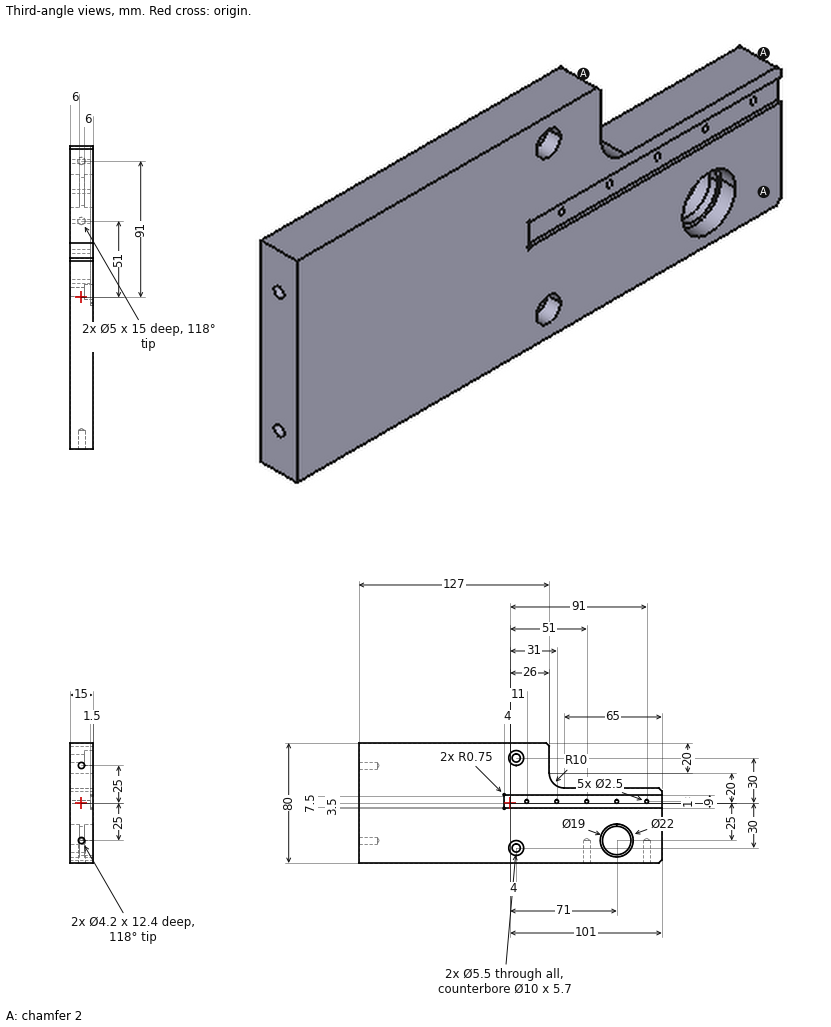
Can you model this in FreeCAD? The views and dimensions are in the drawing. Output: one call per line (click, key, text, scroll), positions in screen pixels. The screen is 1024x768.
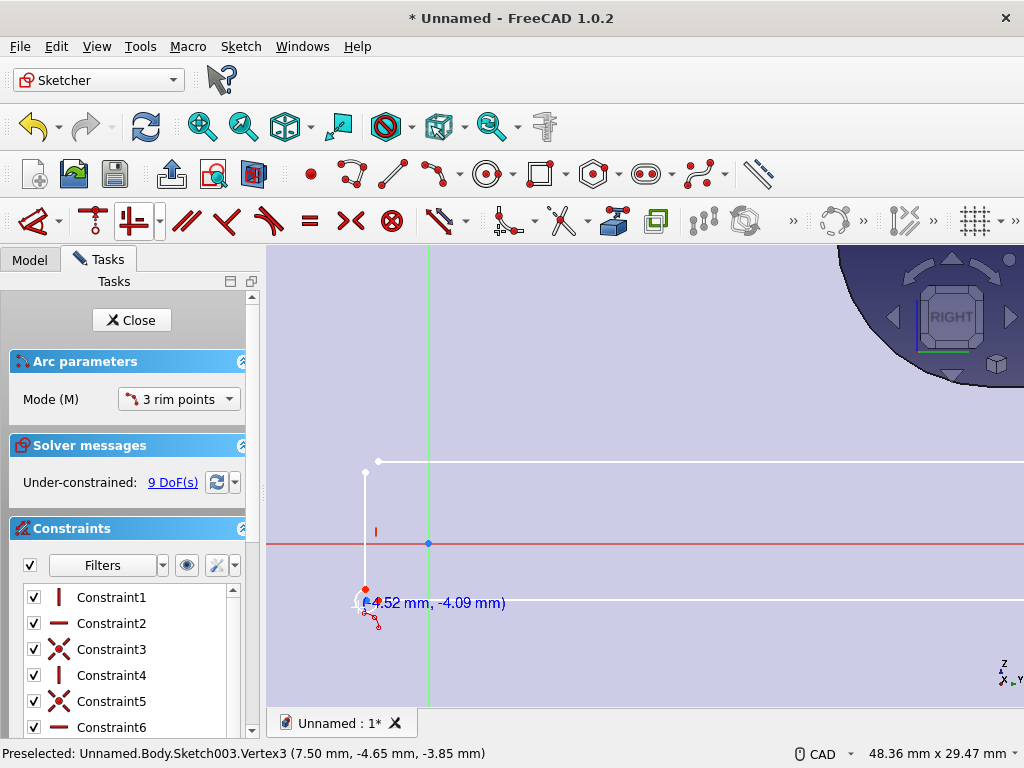
click(378, 462)
click(365, 473)
click(358, 449)
key(Escape)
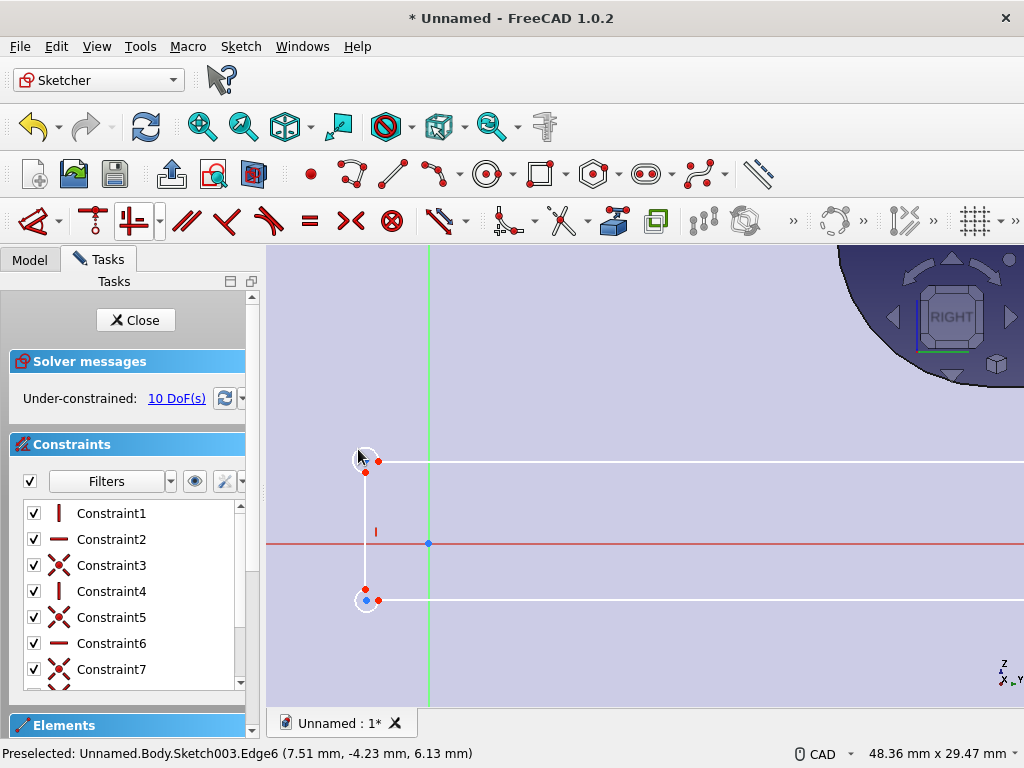
click(355, 600)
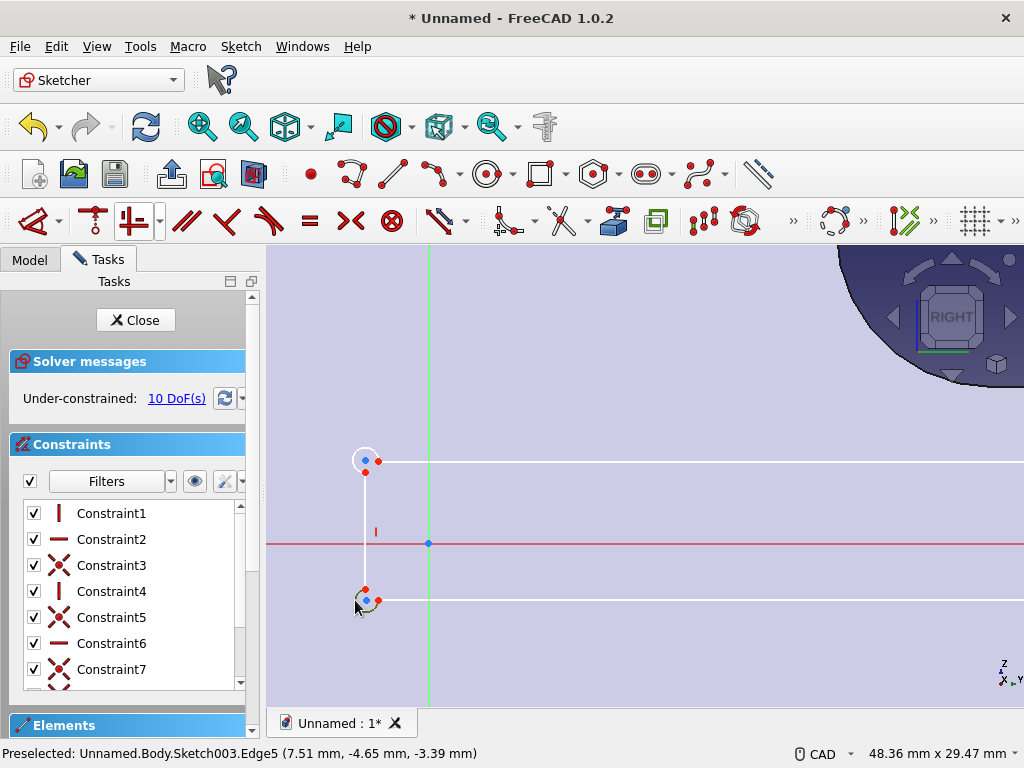
click(369, 448)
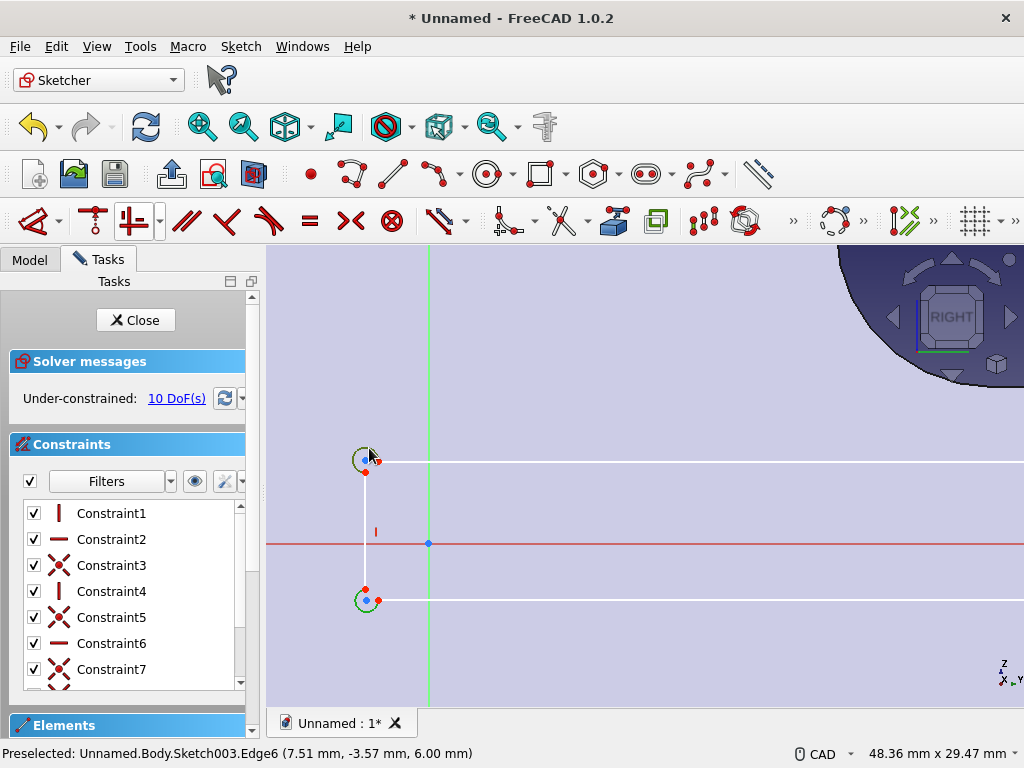
click(310, 222)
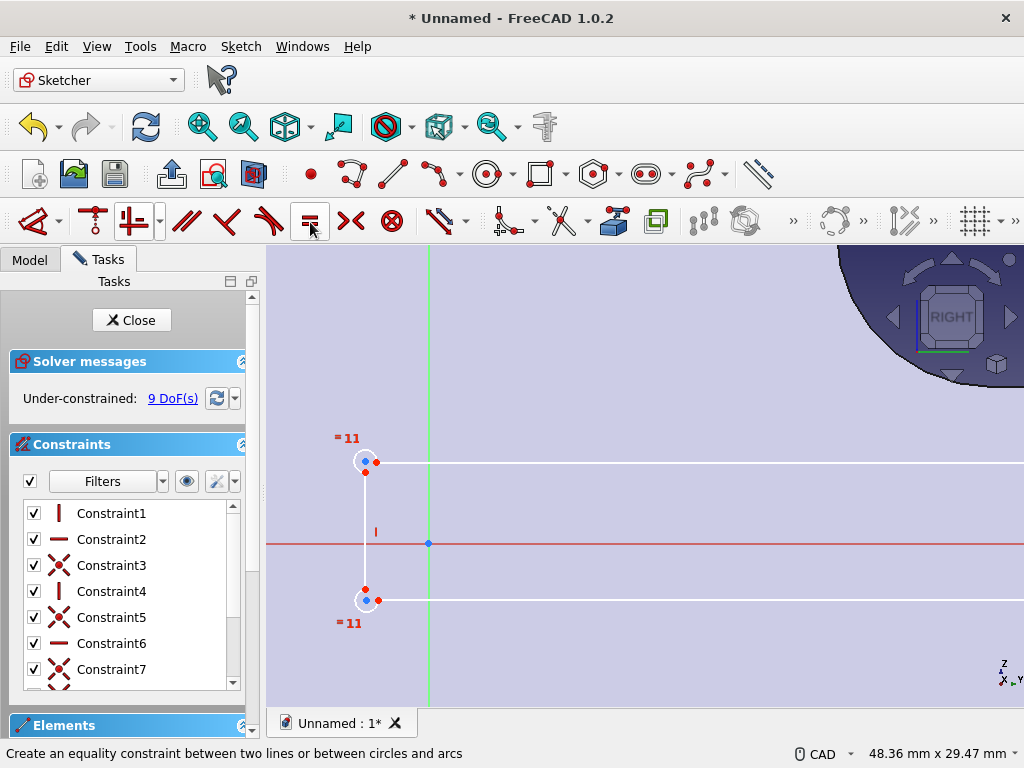
key(d)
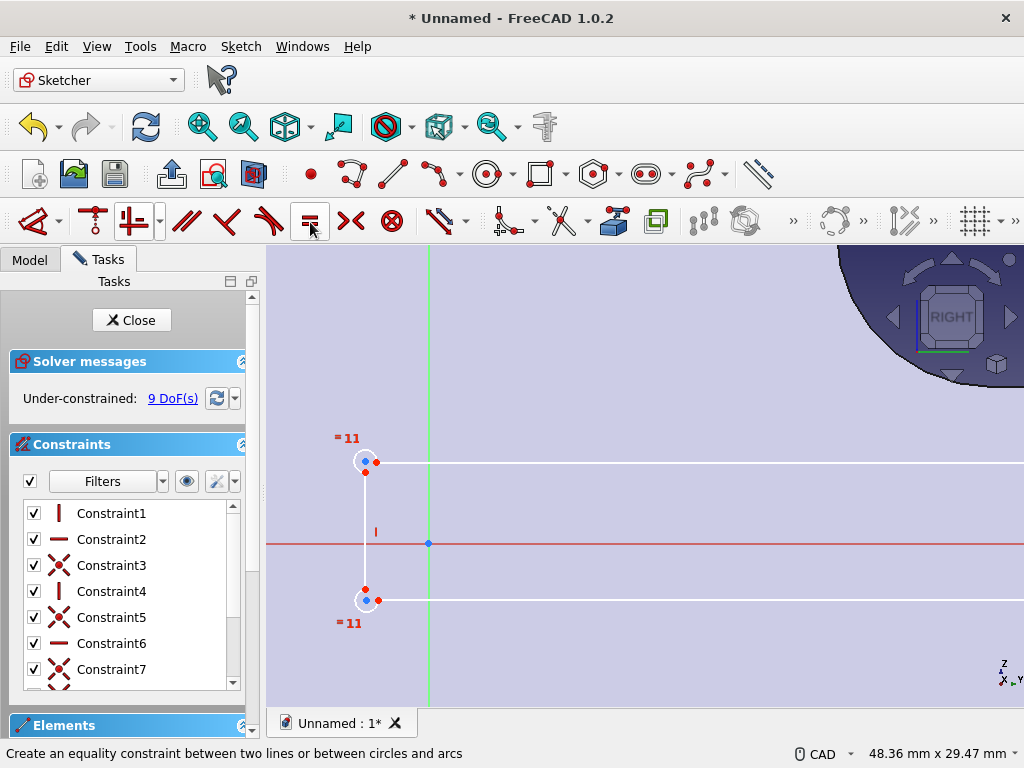
scroll(355, 600, up, 7)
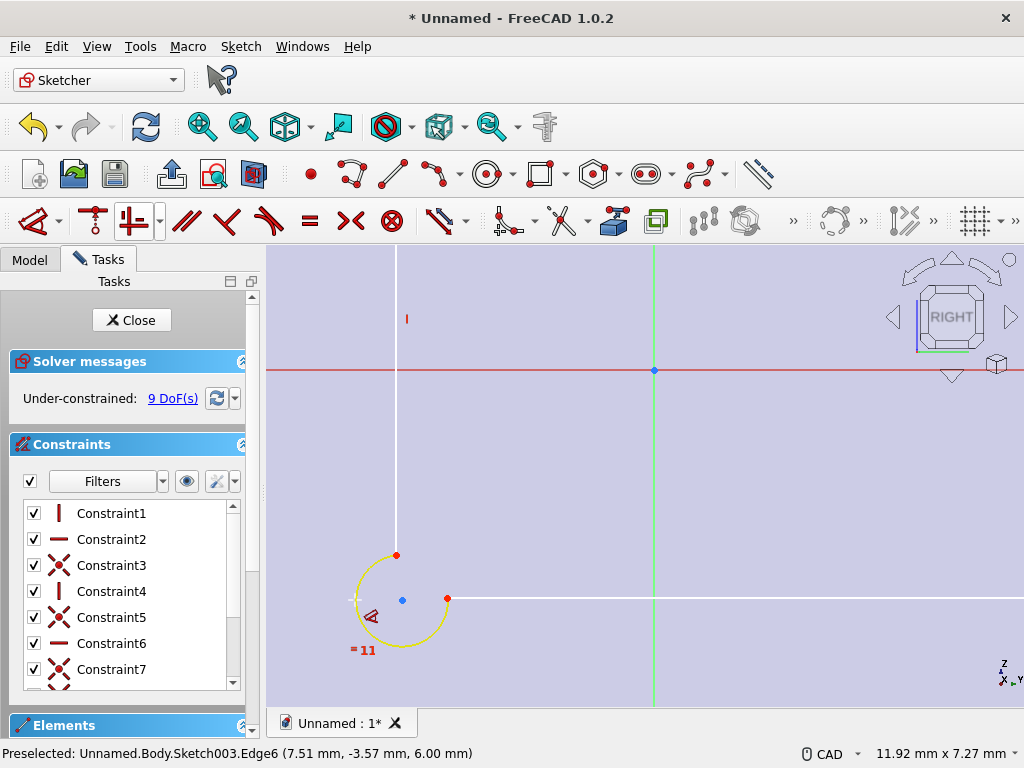
click(356, 599)
click(324, 598)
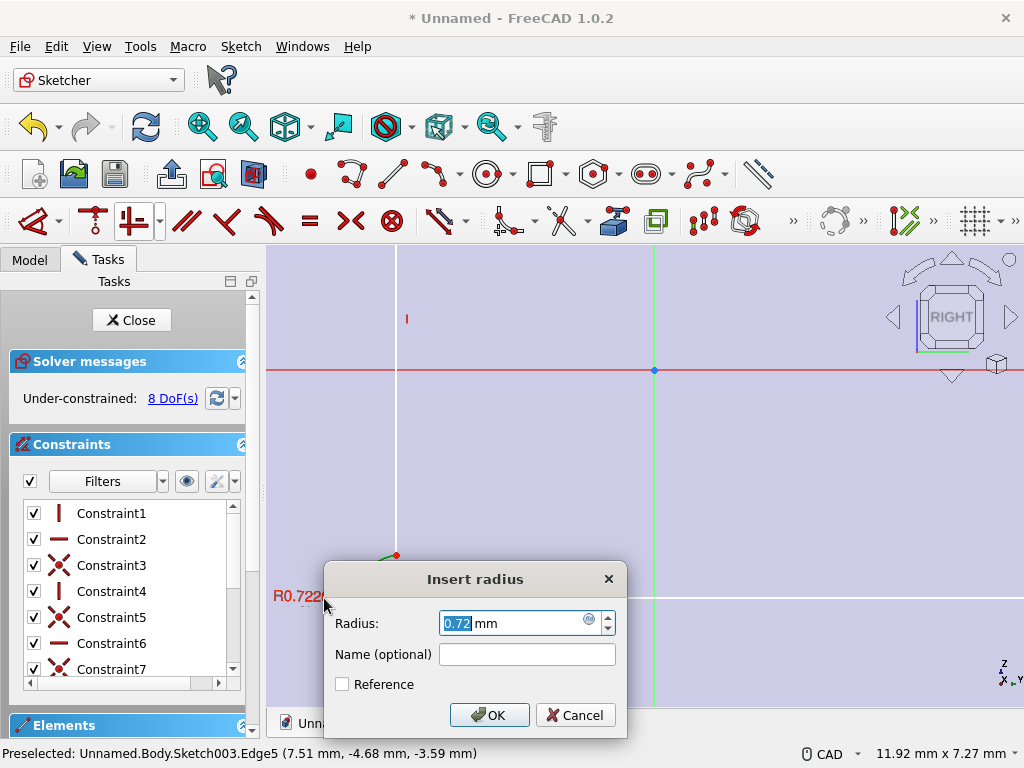
text(0.75)
key(Return)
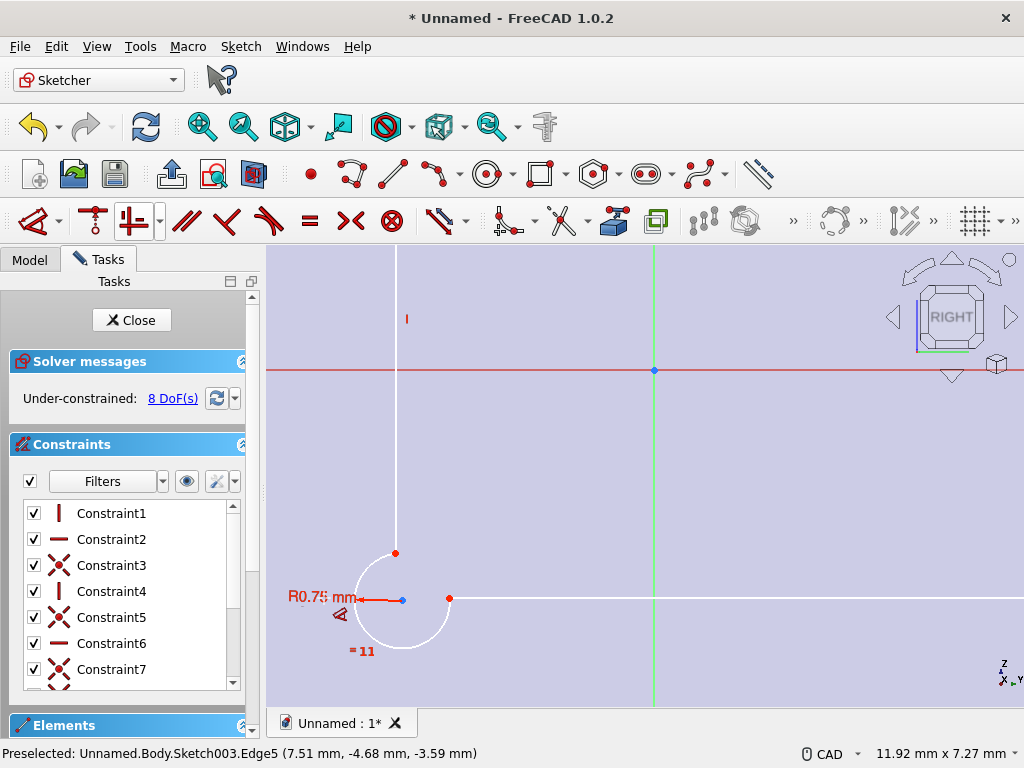
scroll(373, 487, down, 14)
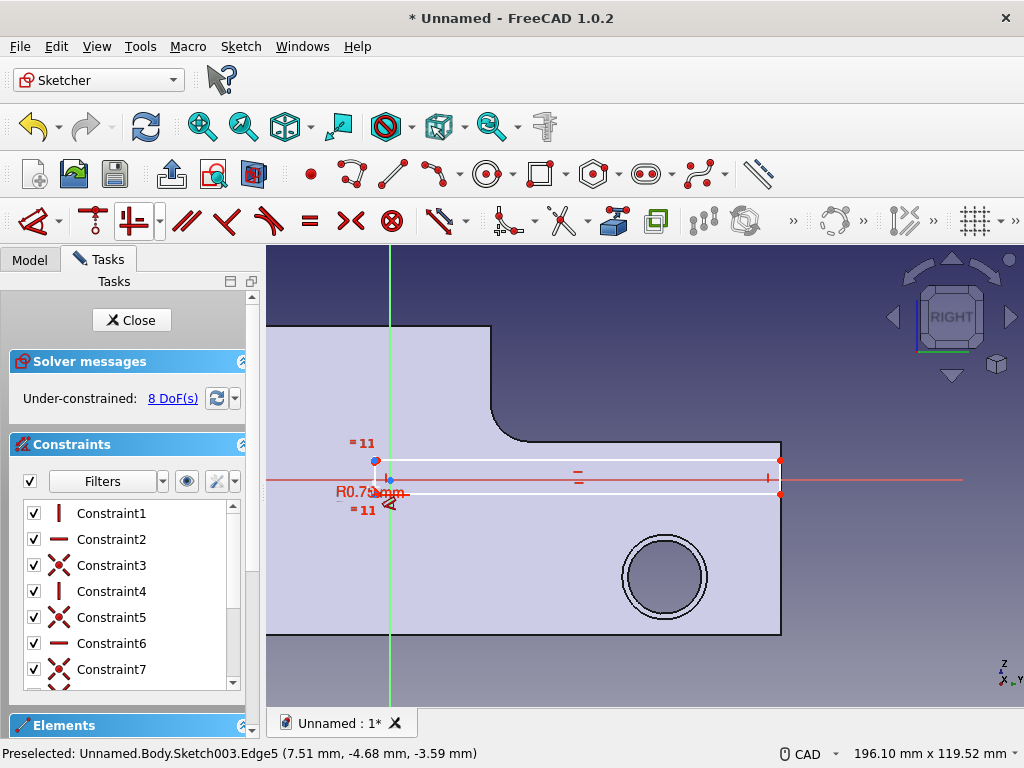
scroll(780, 484, up, 7)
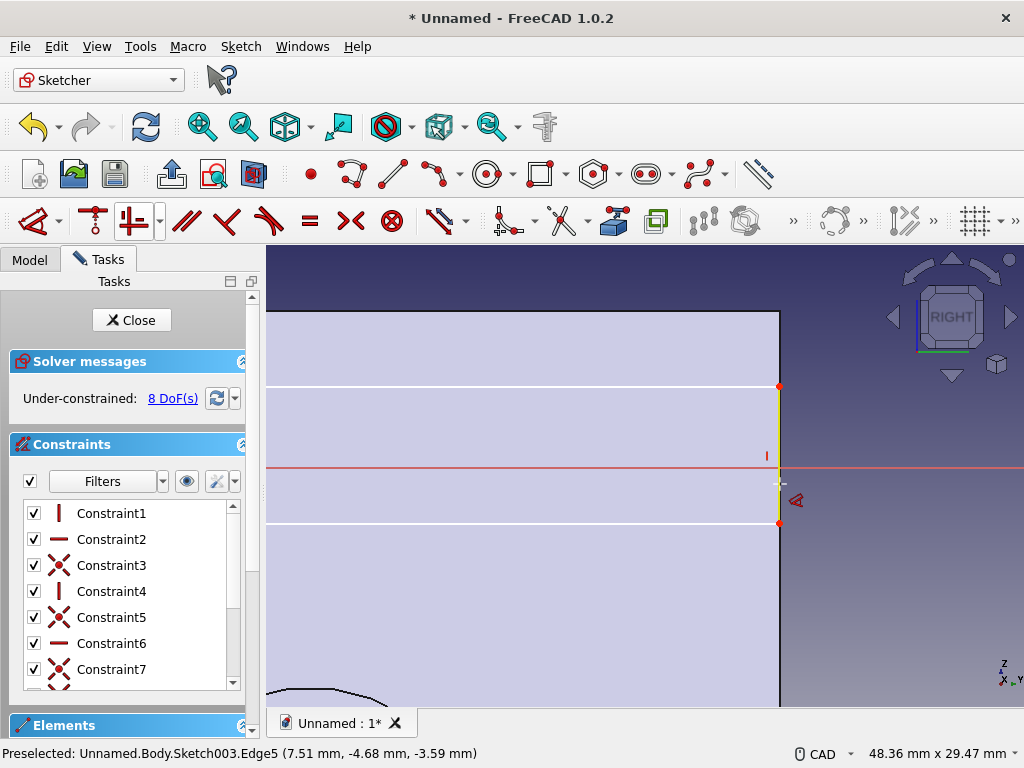
click(779, 483)
click(813, 424)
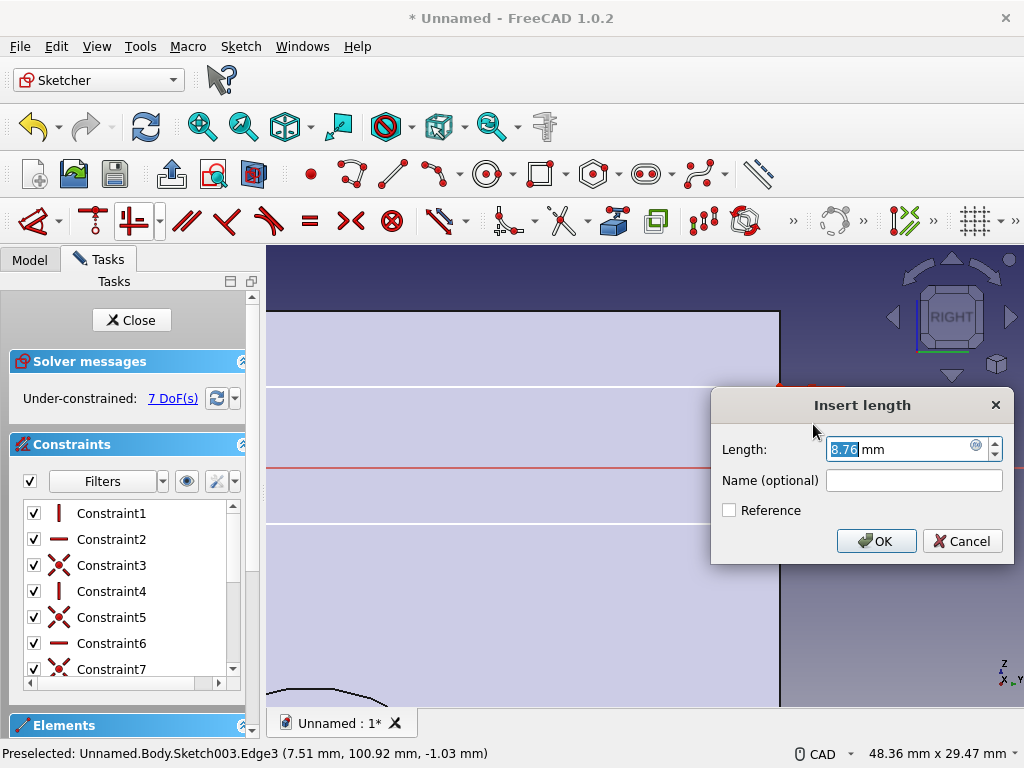
text(9)
key(Return)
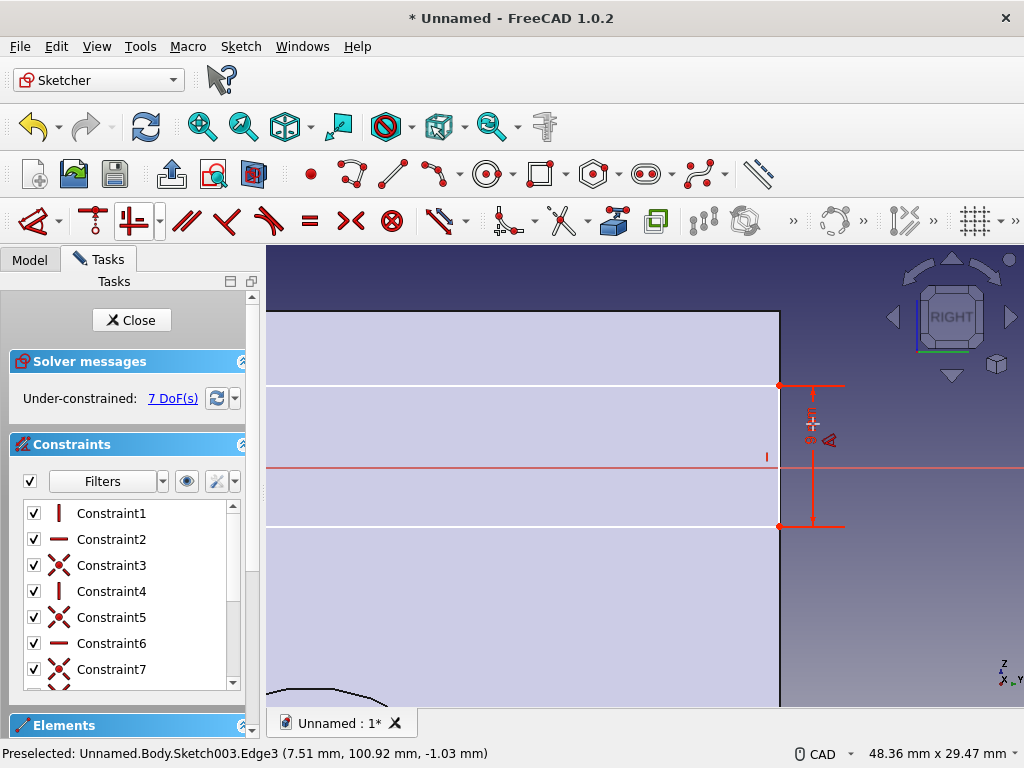
scroll(780, 484, down, 7)